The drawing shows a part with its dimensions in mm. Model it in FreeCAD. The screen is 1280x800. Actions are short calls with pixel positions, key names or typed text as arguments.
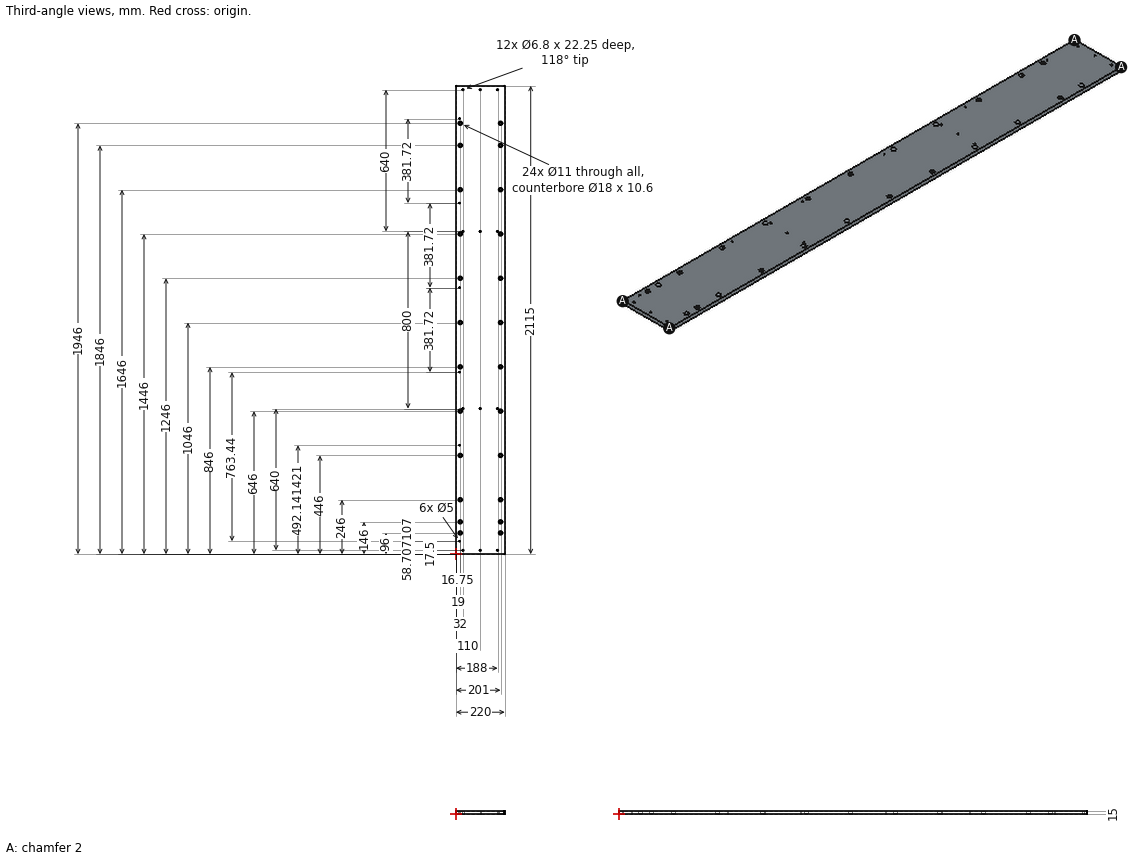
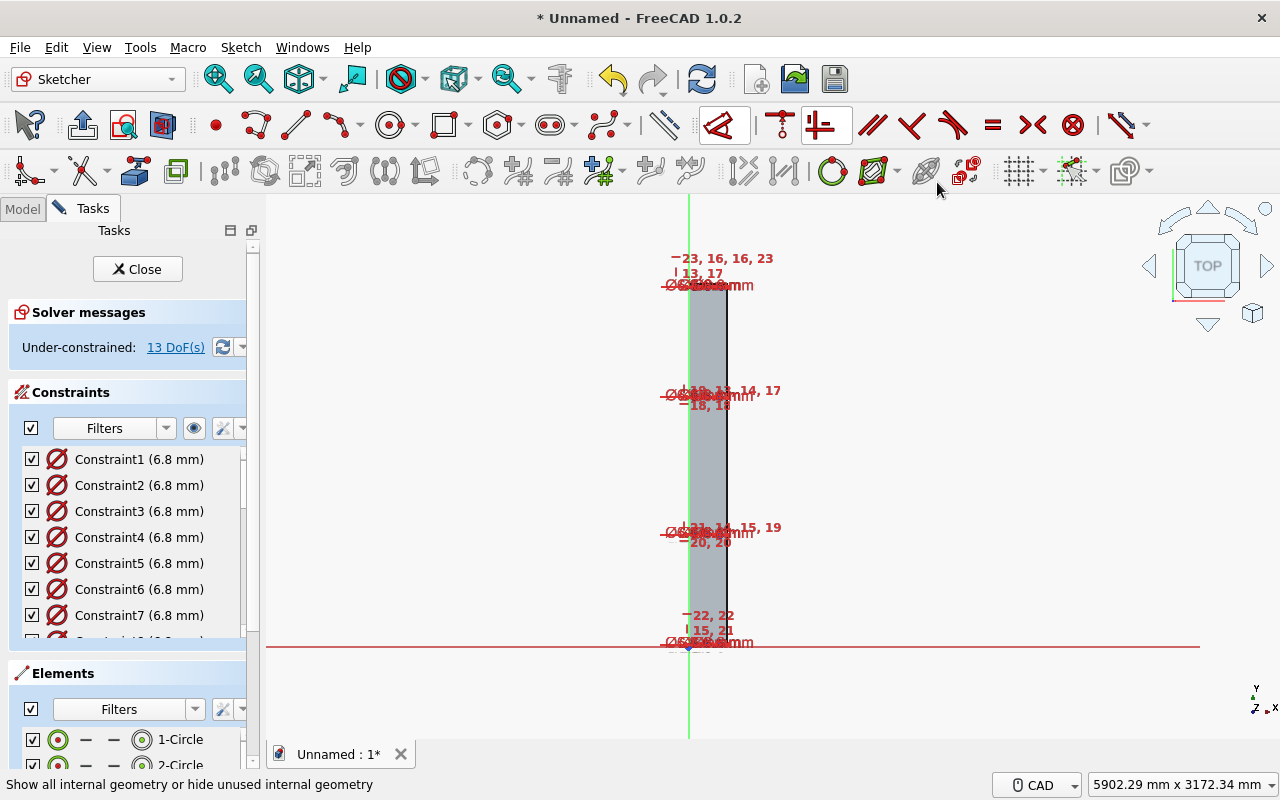
click(721, 287)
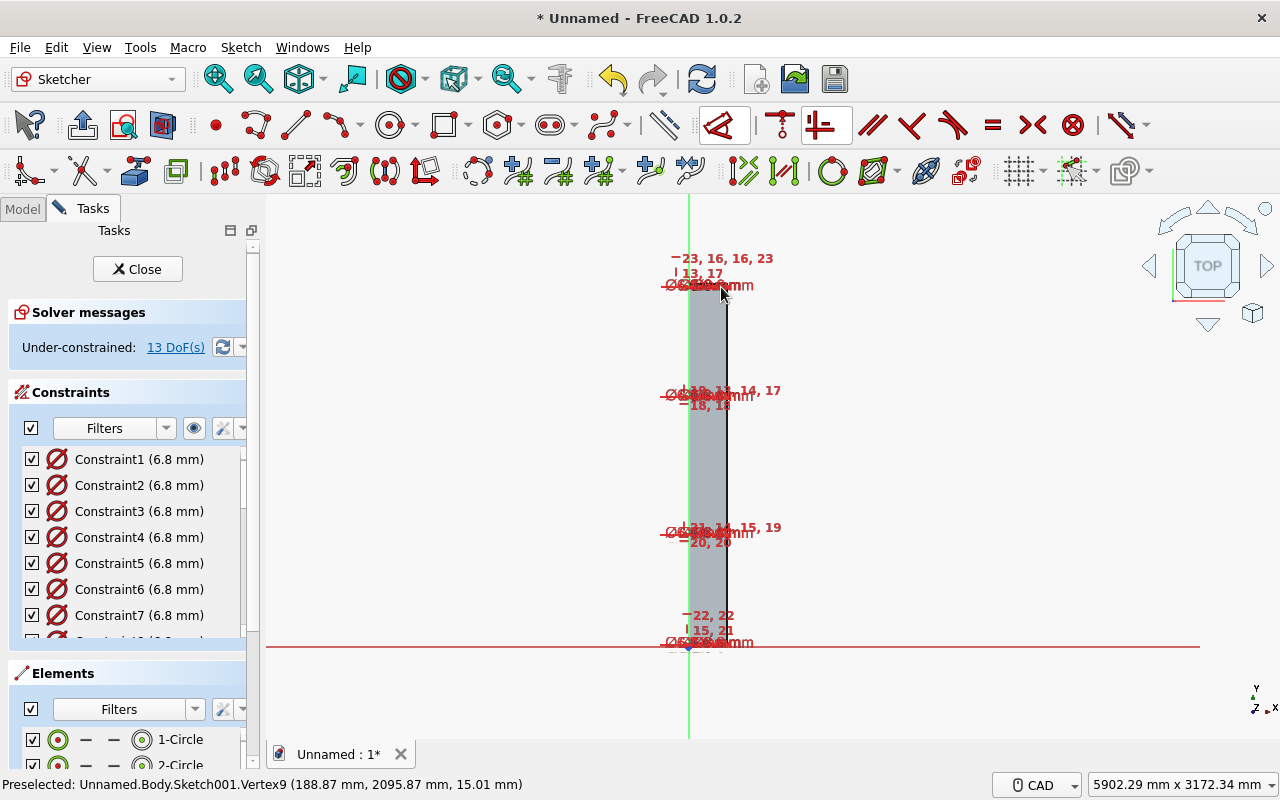
click(721, 398)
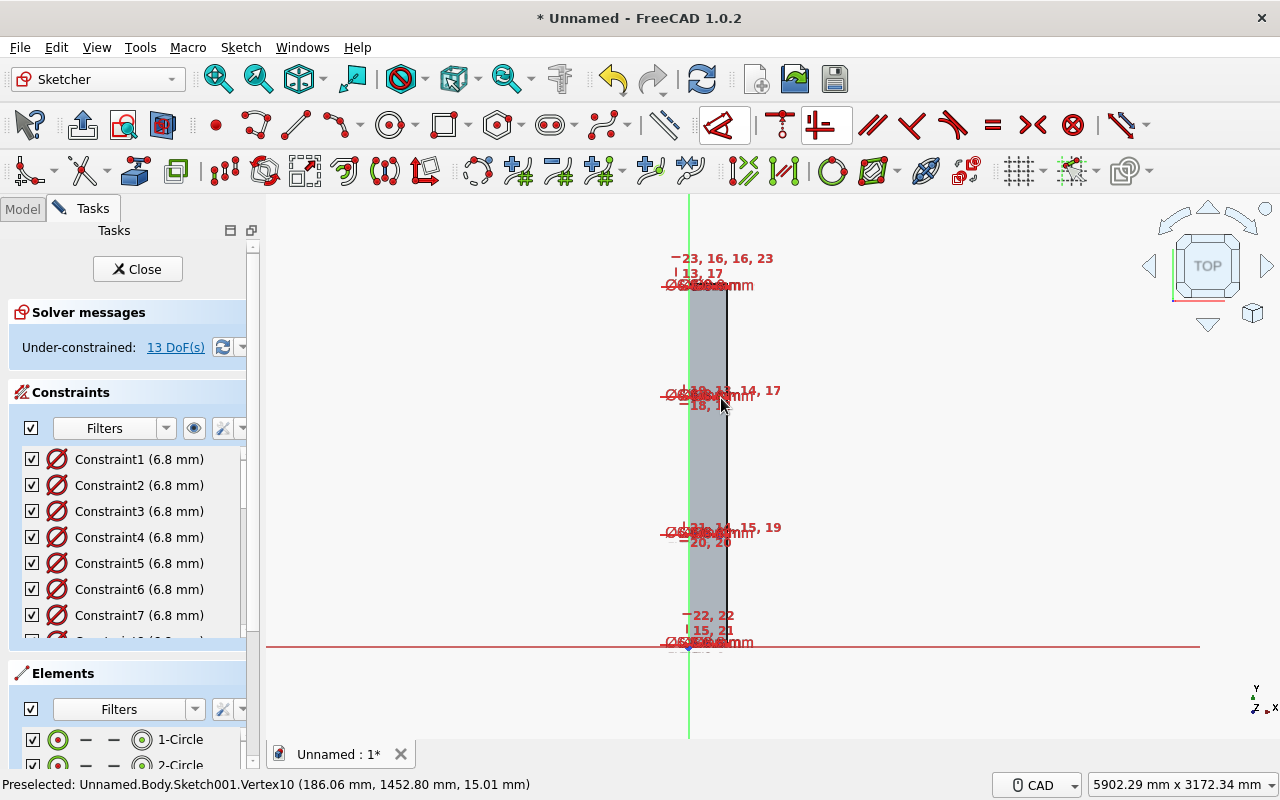
click(846, 126)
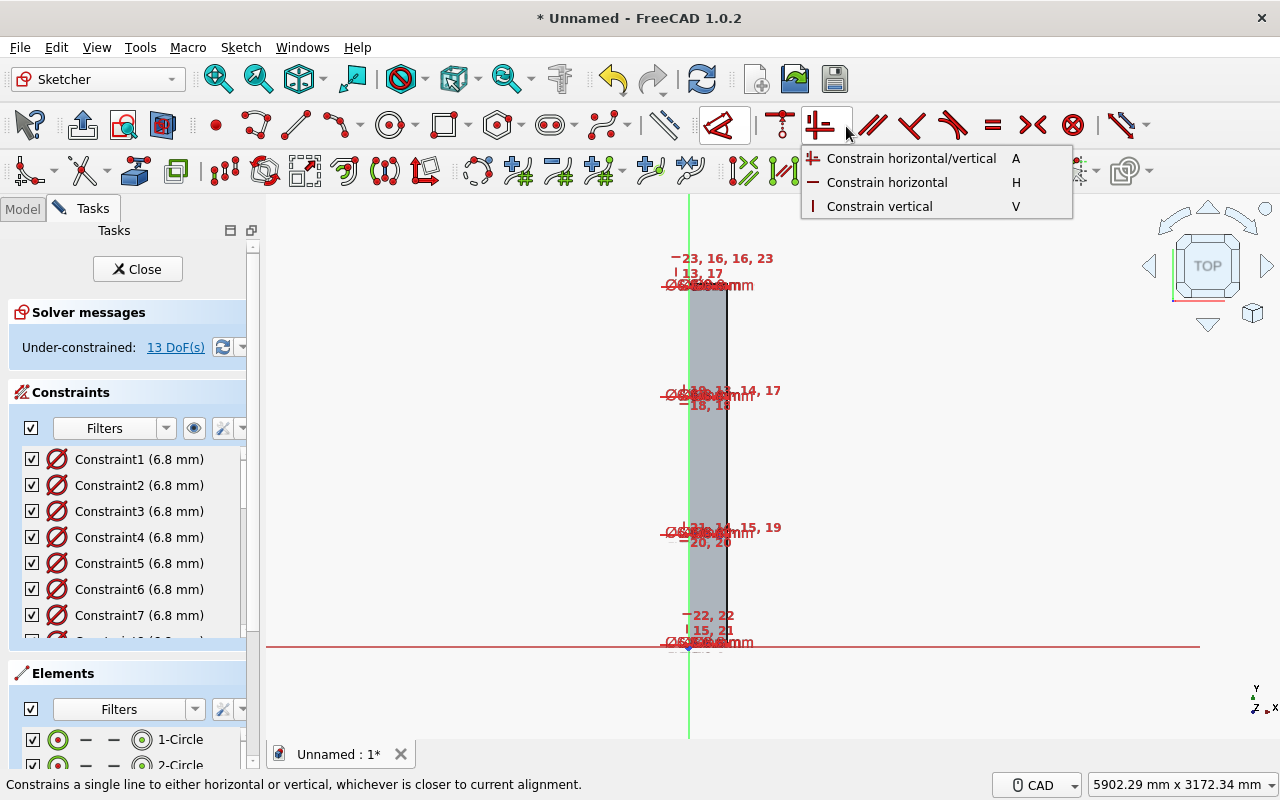
click(937, 206)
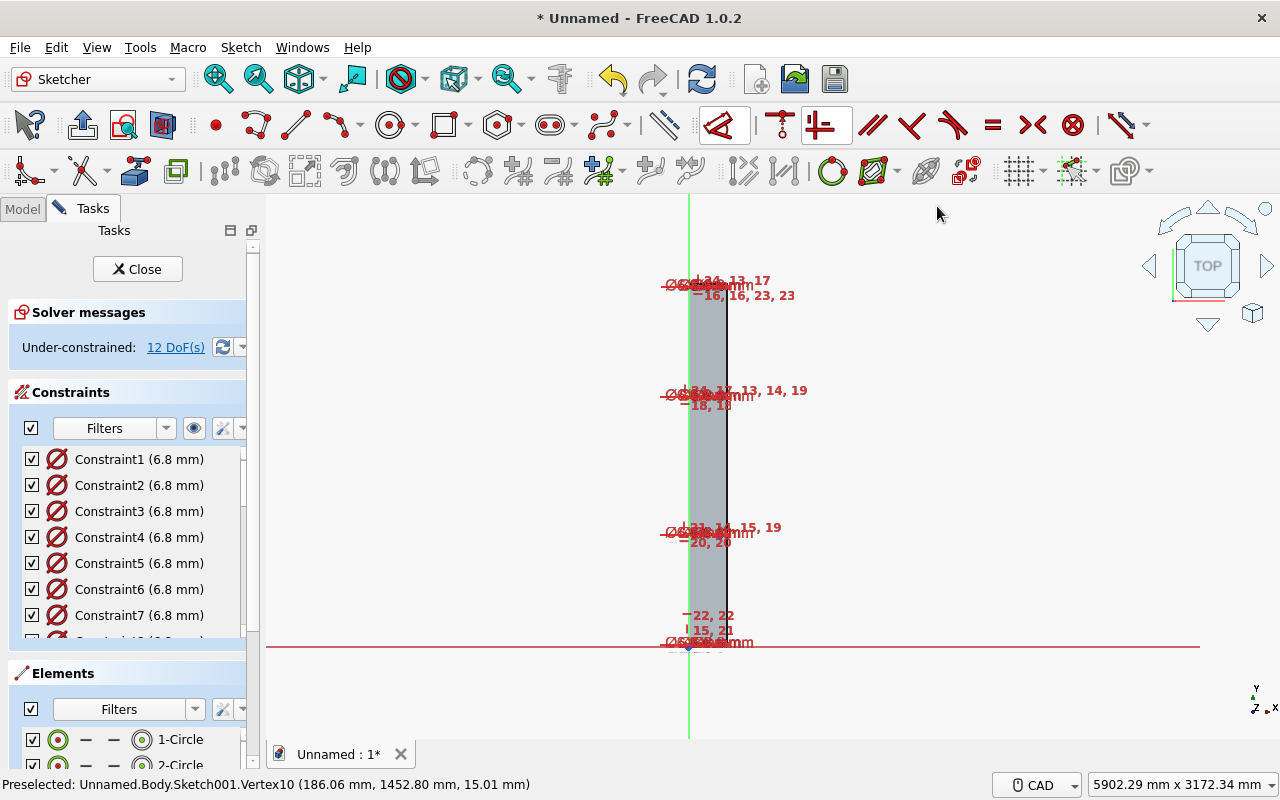
scroll(708, 397, up, 4)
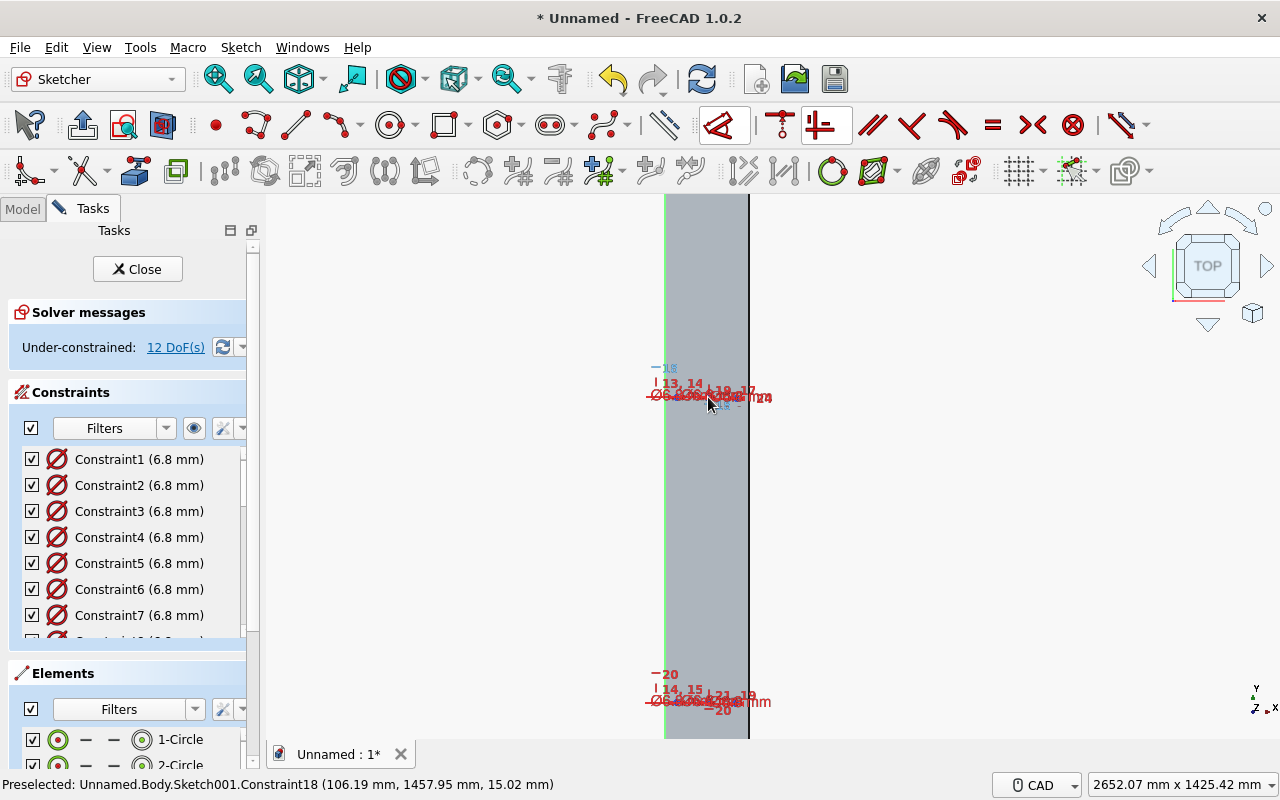
click(707, 397)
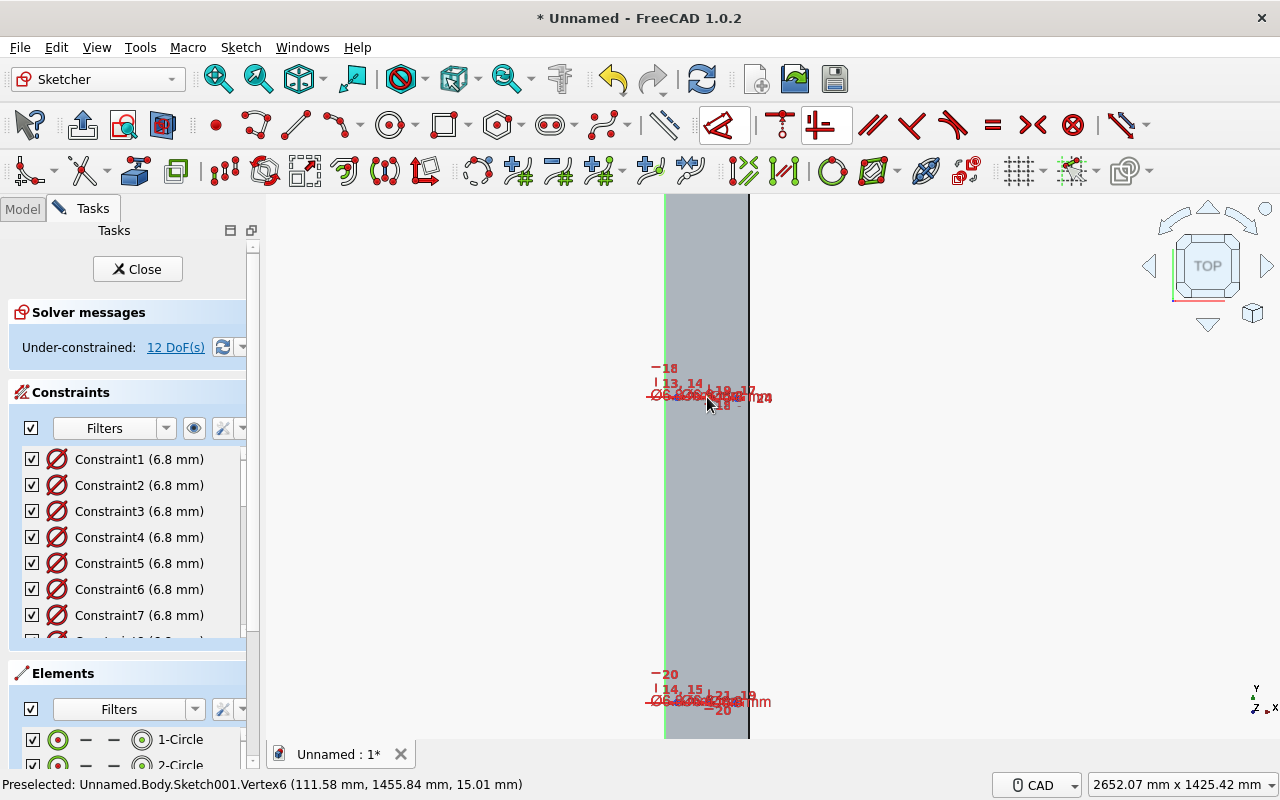
click(737, 399)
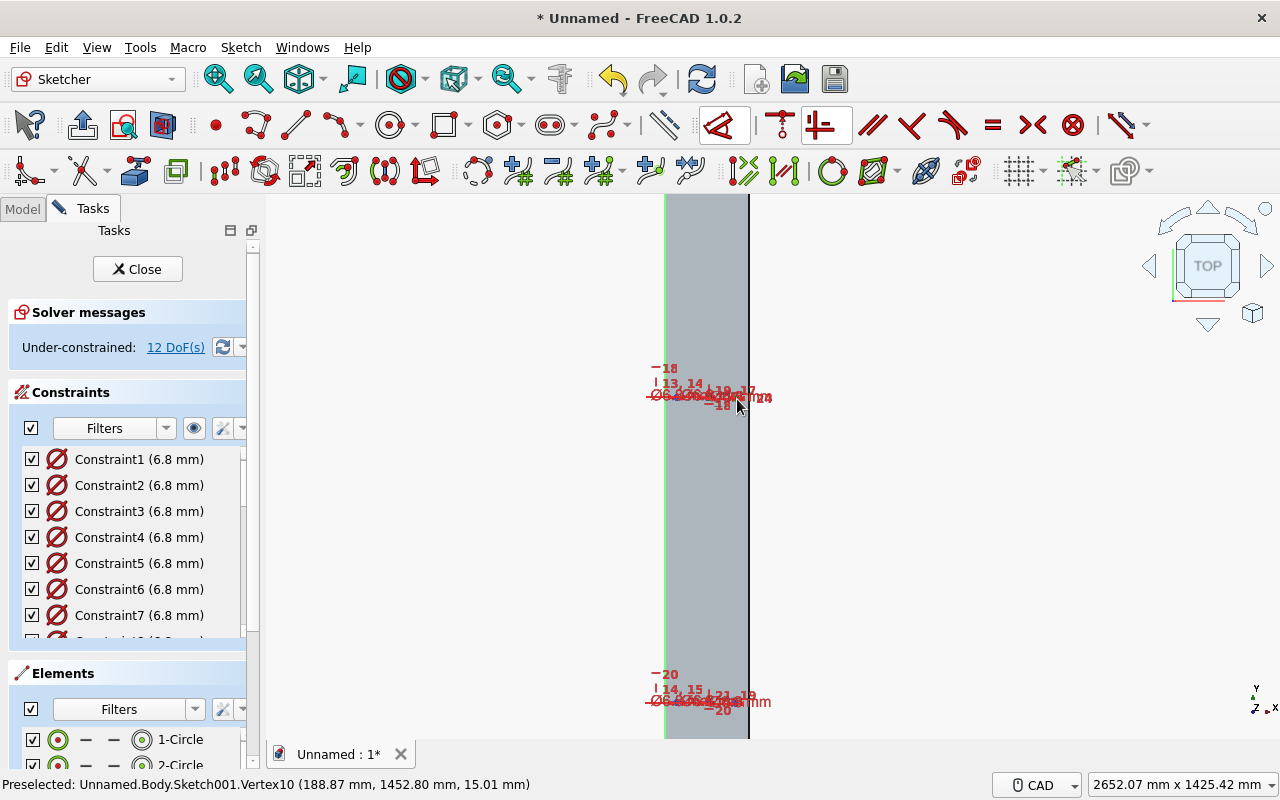
key(h)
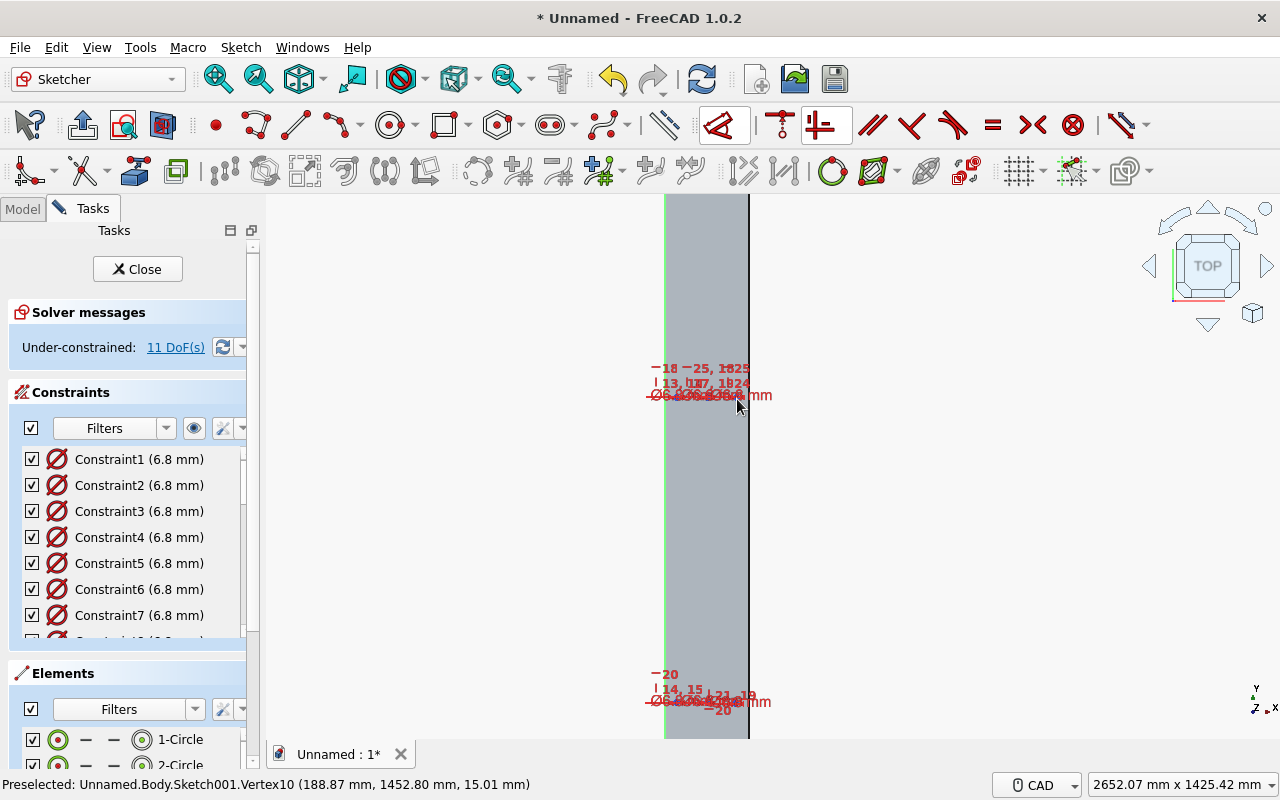
click(737, 397)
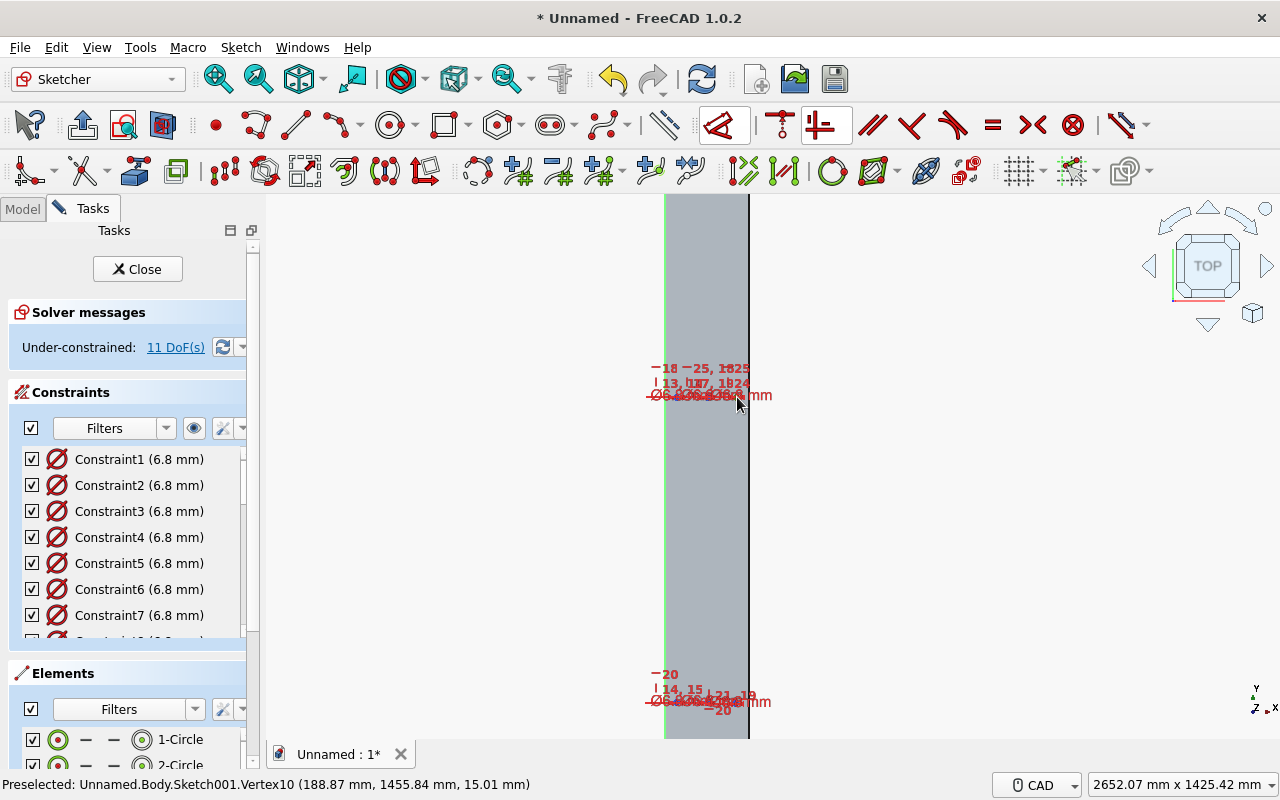
click(736, 704)